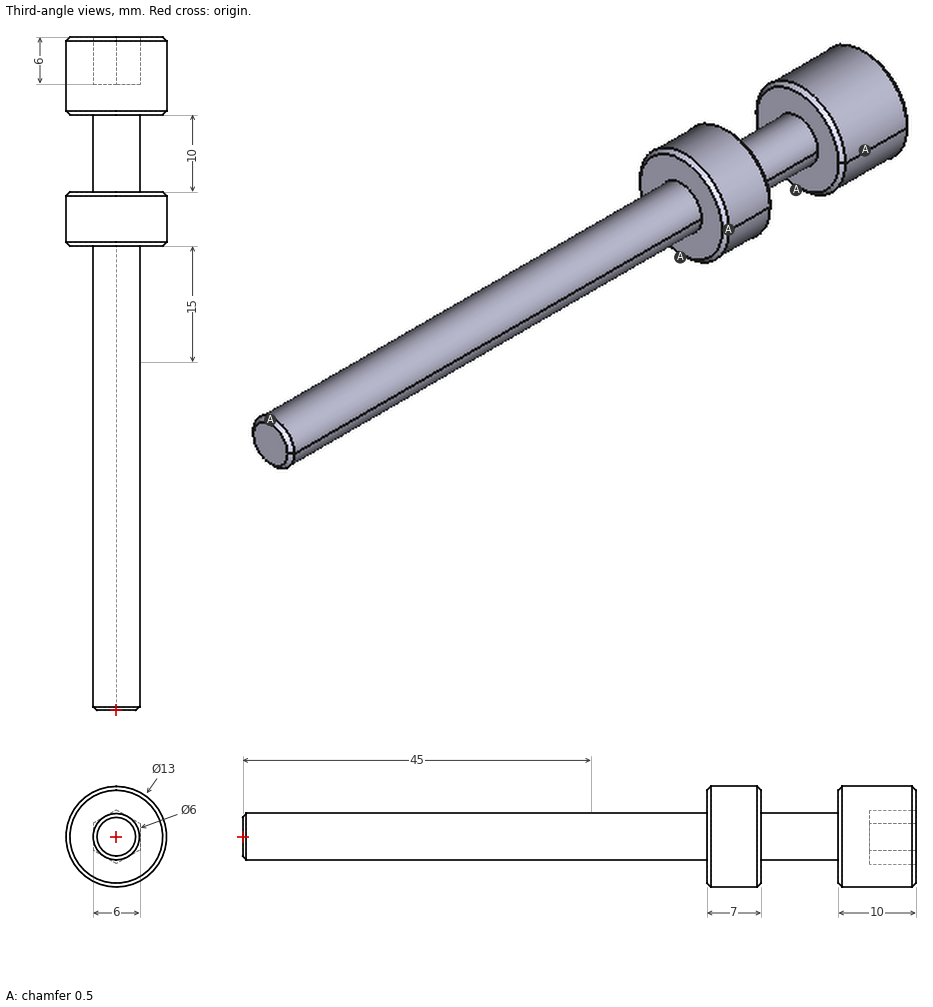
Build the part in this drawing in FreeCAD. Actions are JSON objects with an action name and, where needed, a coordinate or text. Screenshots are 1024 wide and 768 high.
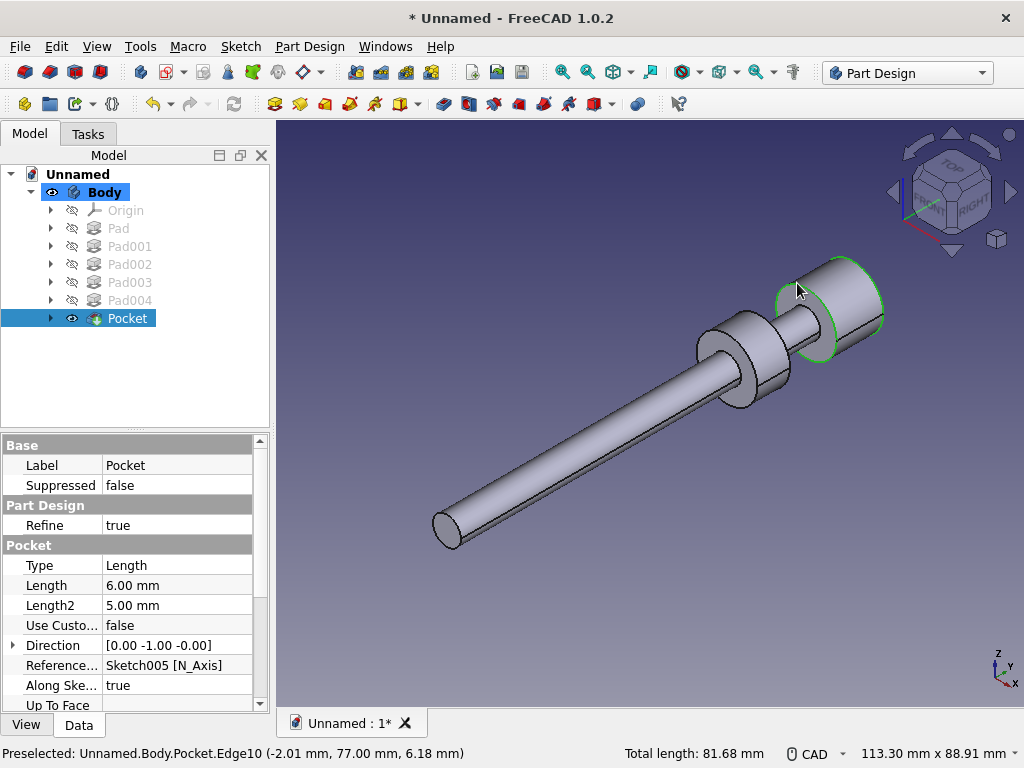
{"action": "left_click", "coordinate": [436, 514], "text": "ctrl"}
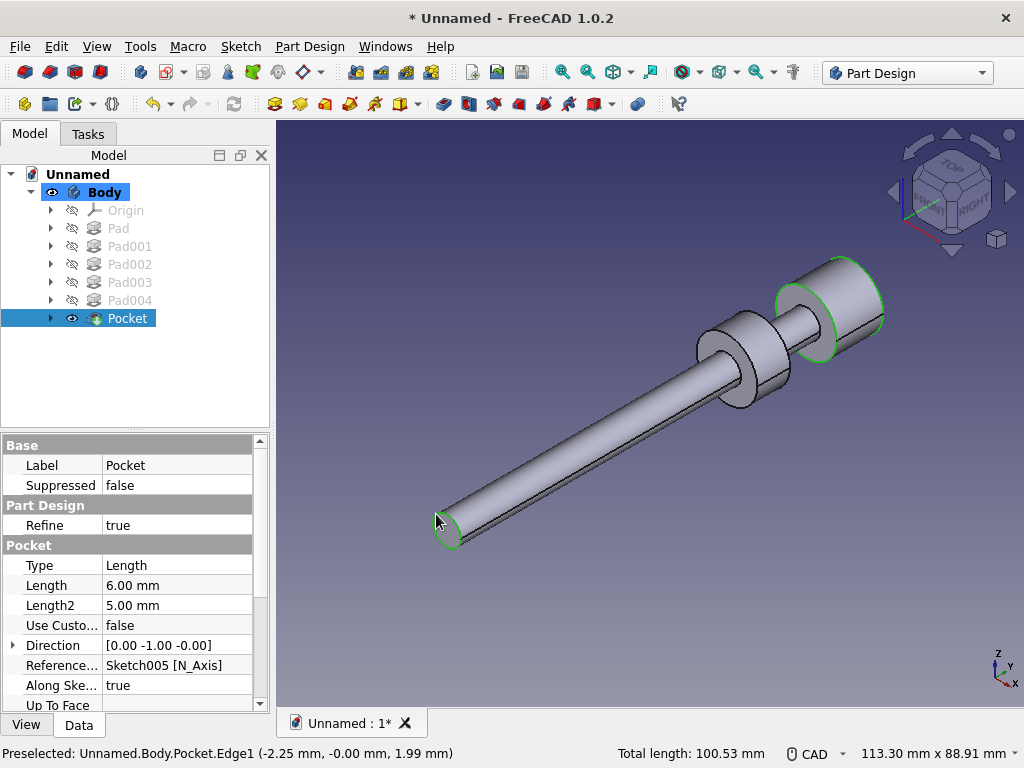
{"action": "left_click", "coordinate": [718, 329], "text": "ctrl"}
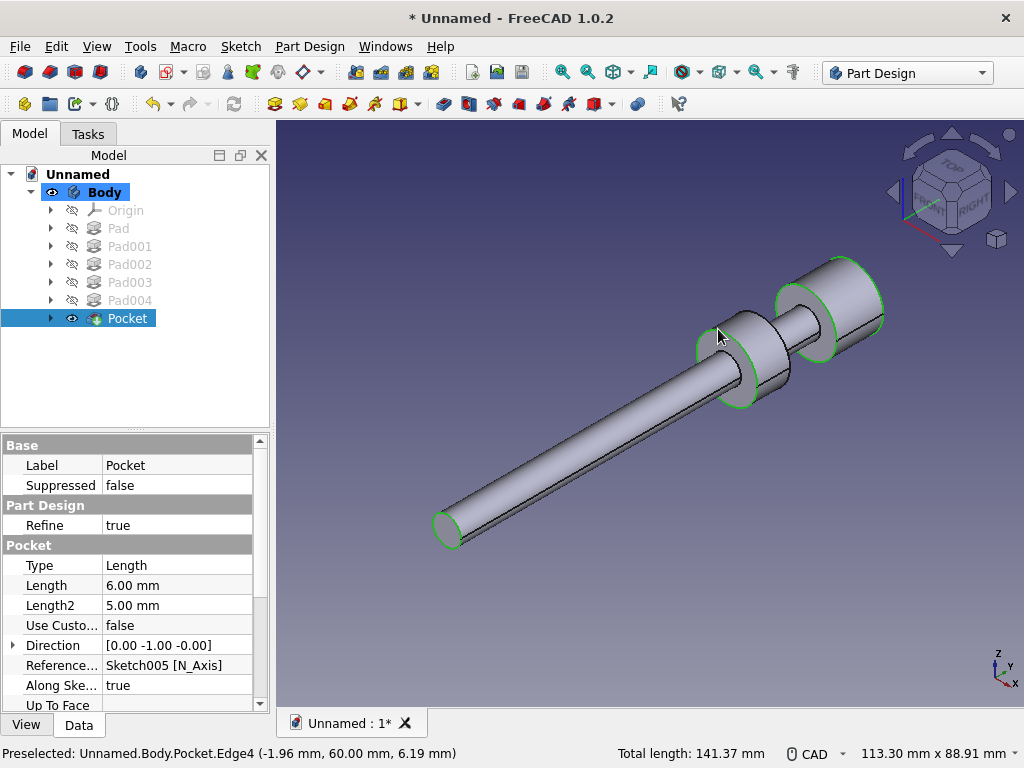
{"action": "key", "text": "2"}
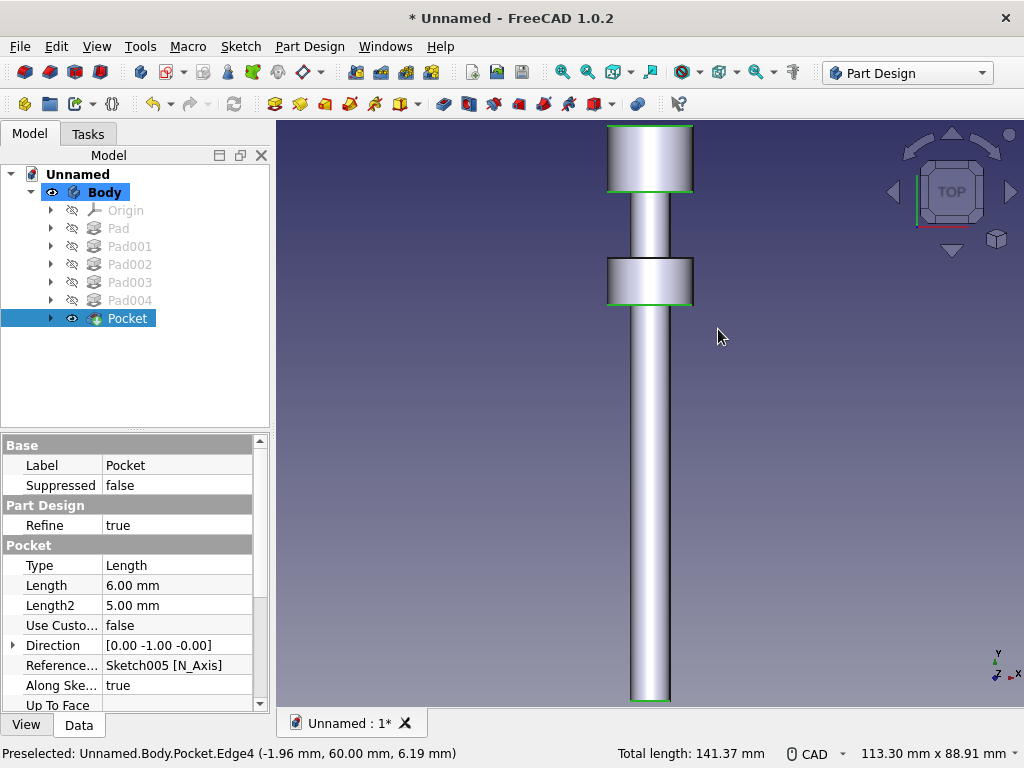
{"action": "left_click", "coordinate": [615, 257], "text": "ctrl"}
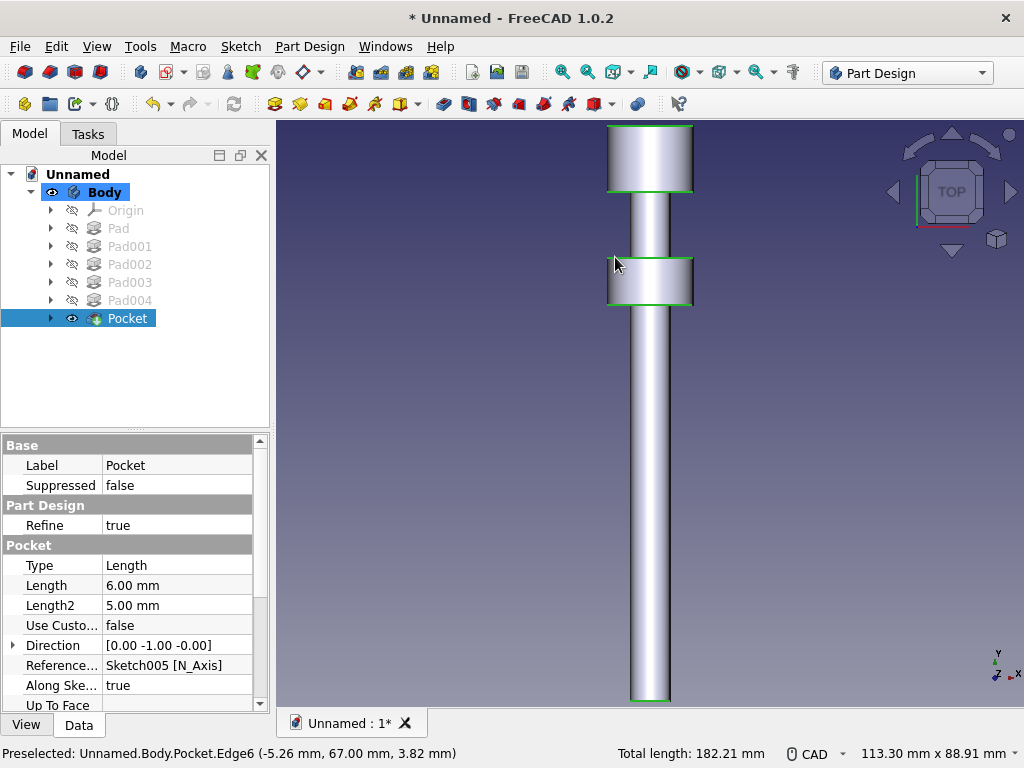
{"action": "left_click", "coordinate": [50, 72]}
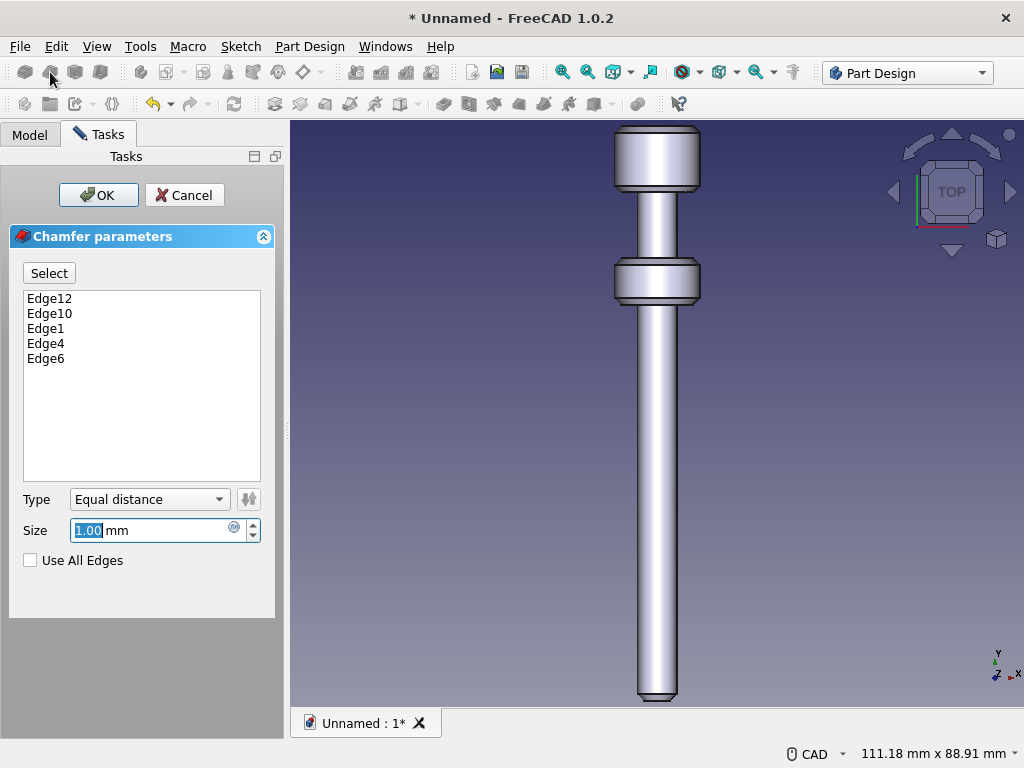
{"action": "type", "text": "0.5"}
{"action": "key", "text": "Tab"}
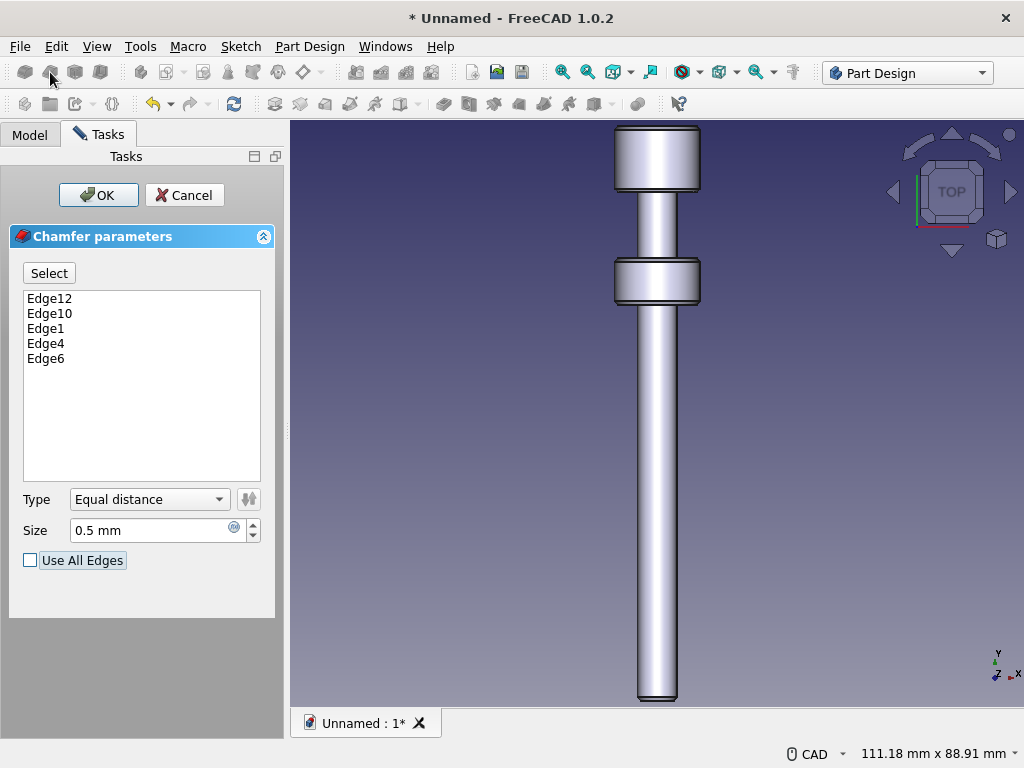
{"action": "left_click", "coordinate": [99, 195]}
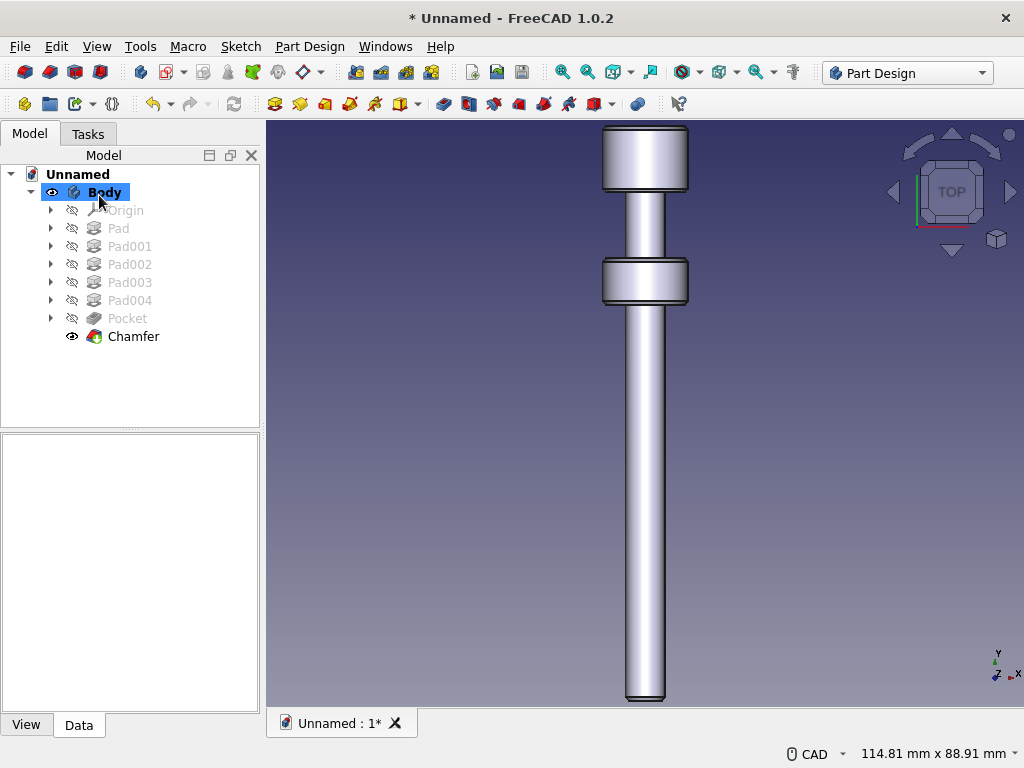
{"action": "key", "text": "0"}